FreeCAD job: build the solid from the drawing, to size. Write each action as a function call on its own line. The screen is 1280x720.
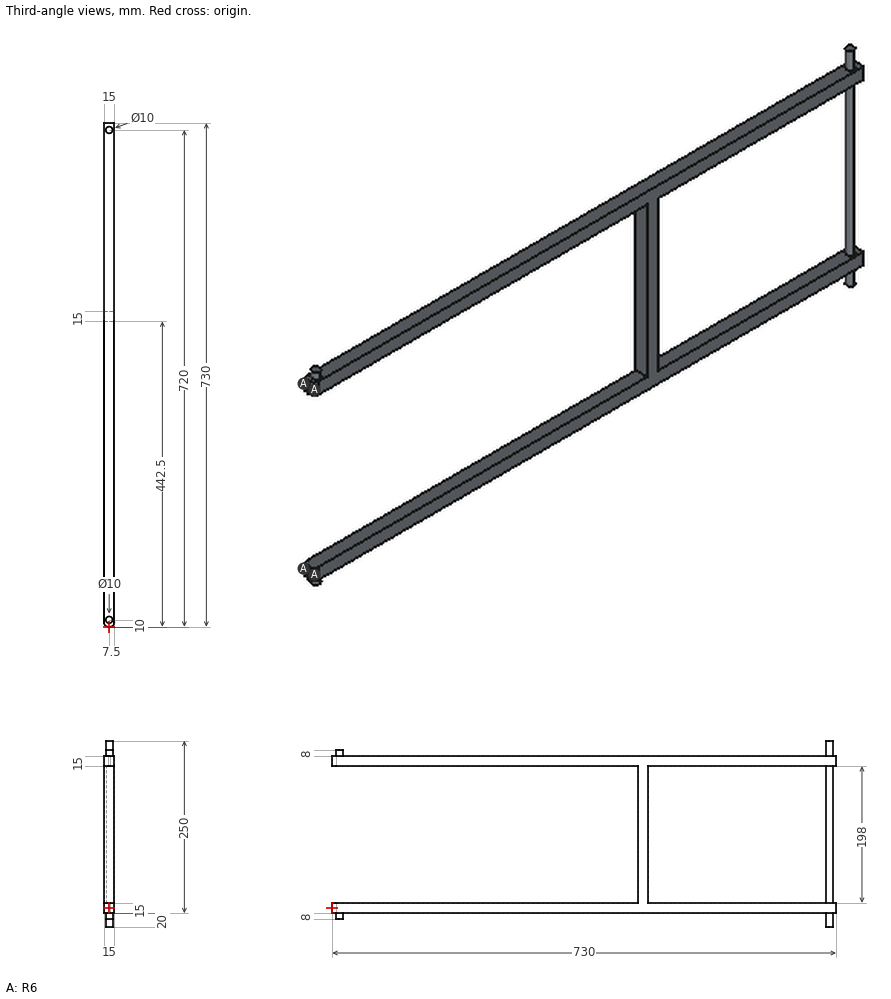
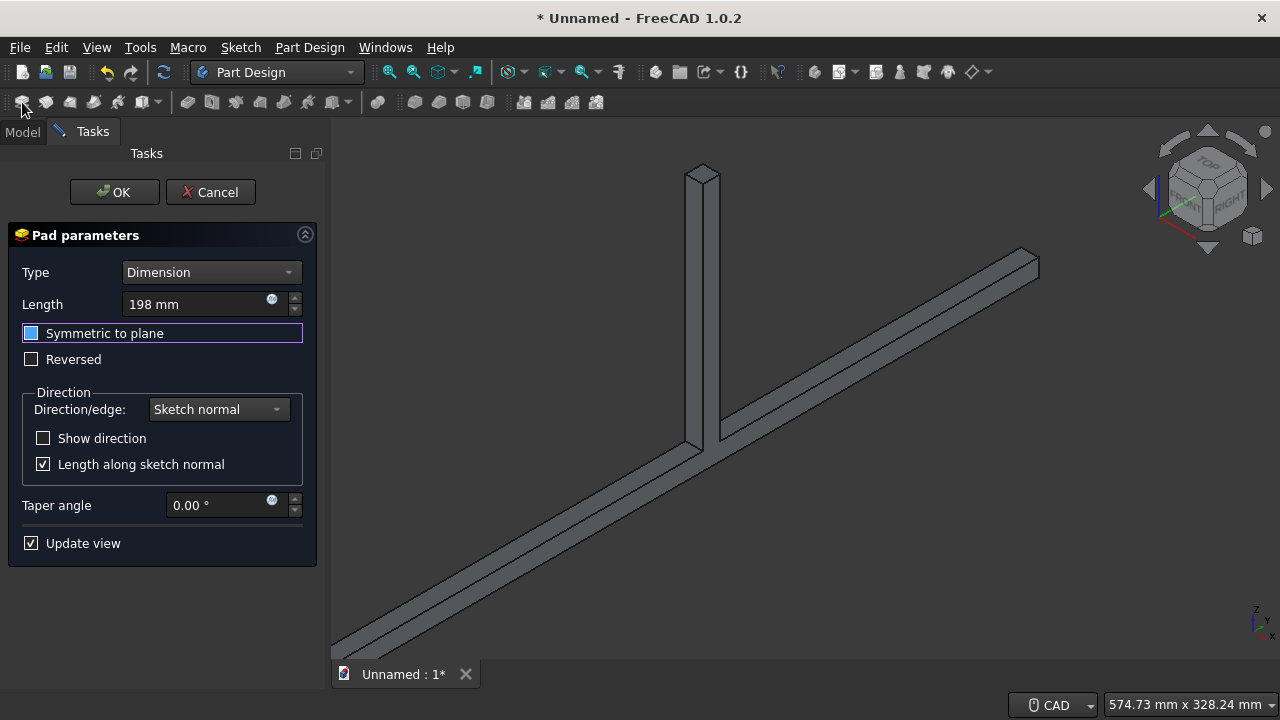
click(115, 192)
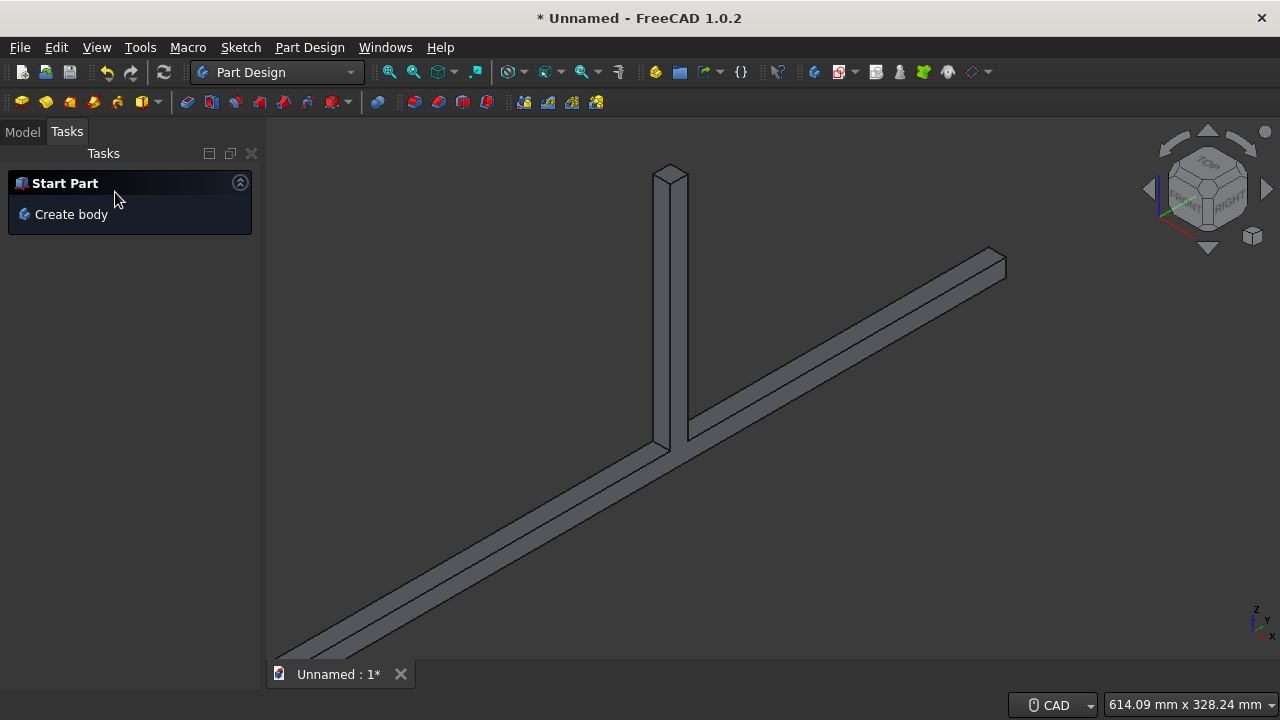
click(390, 72)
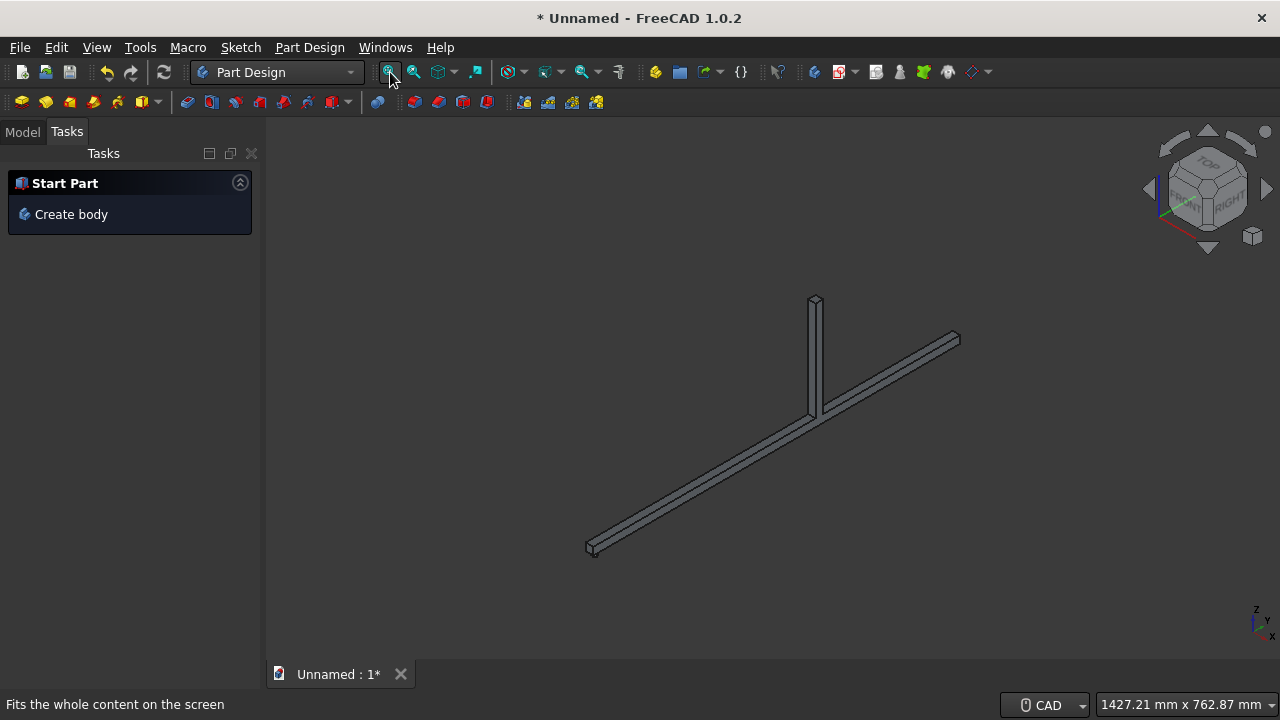
scroll(816, 298, up, 5)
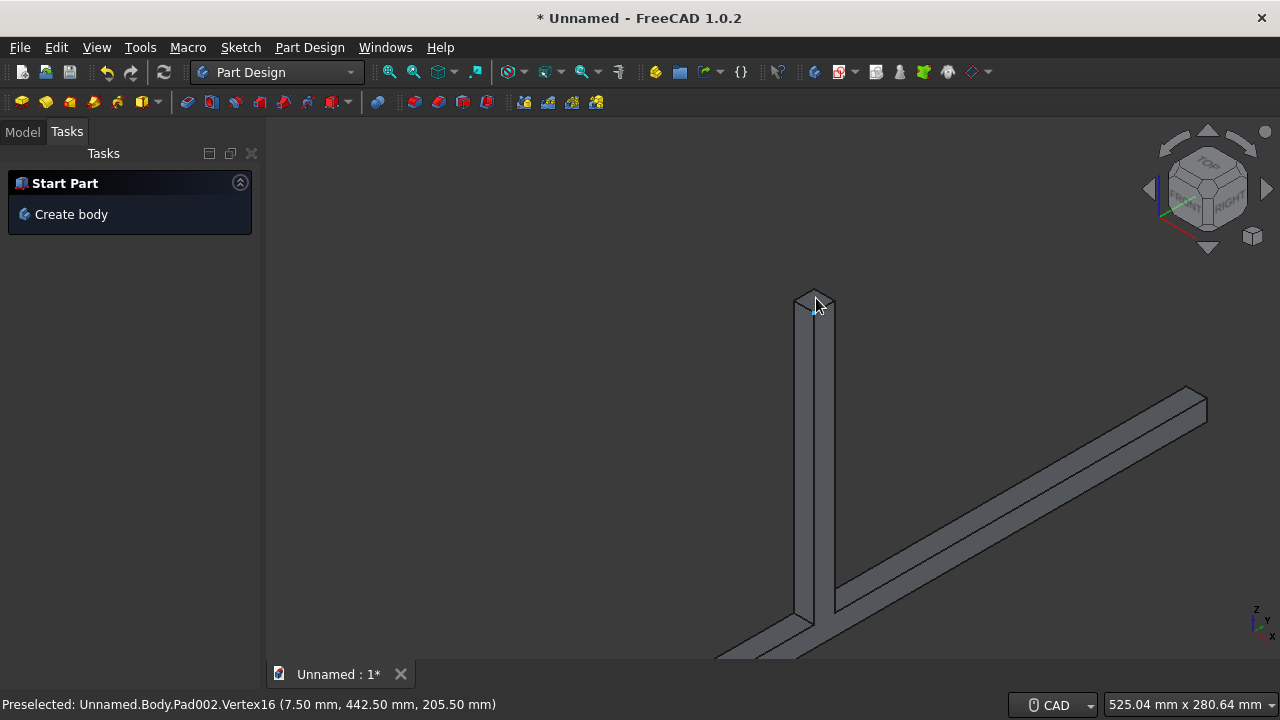
click(814, 300)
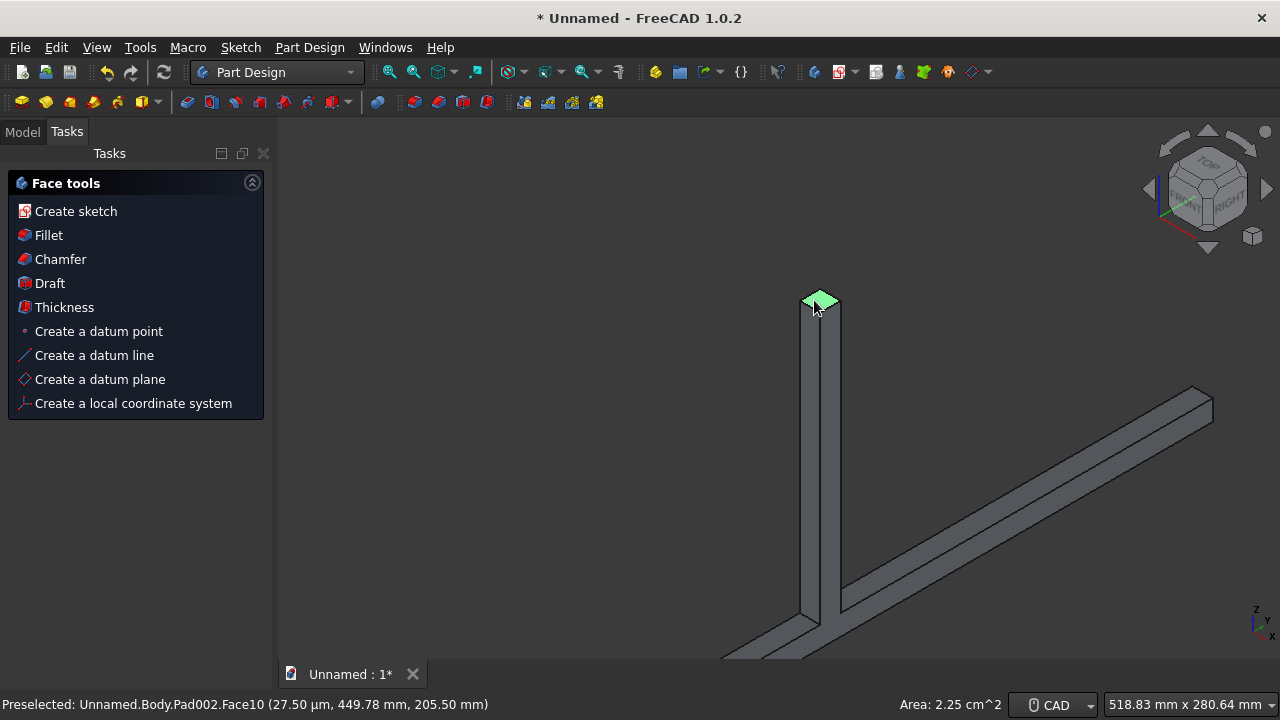
click(840, 72)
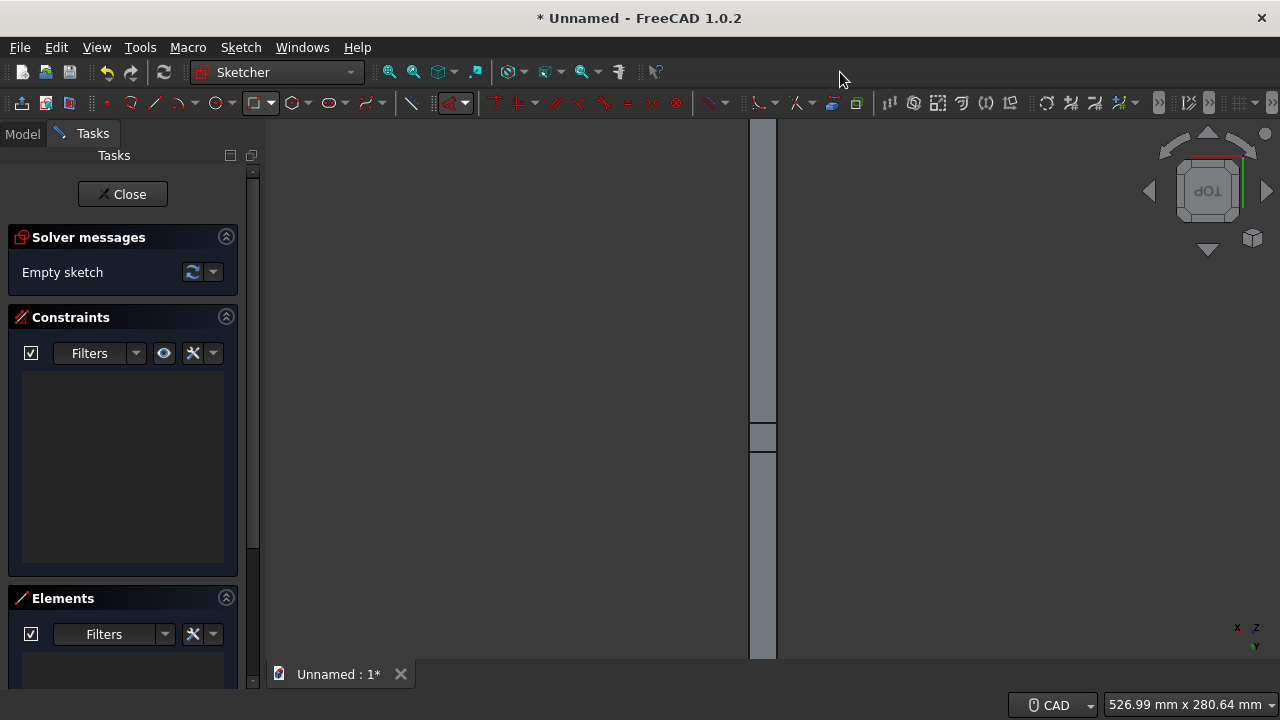
scroll(685, 427, down, 7)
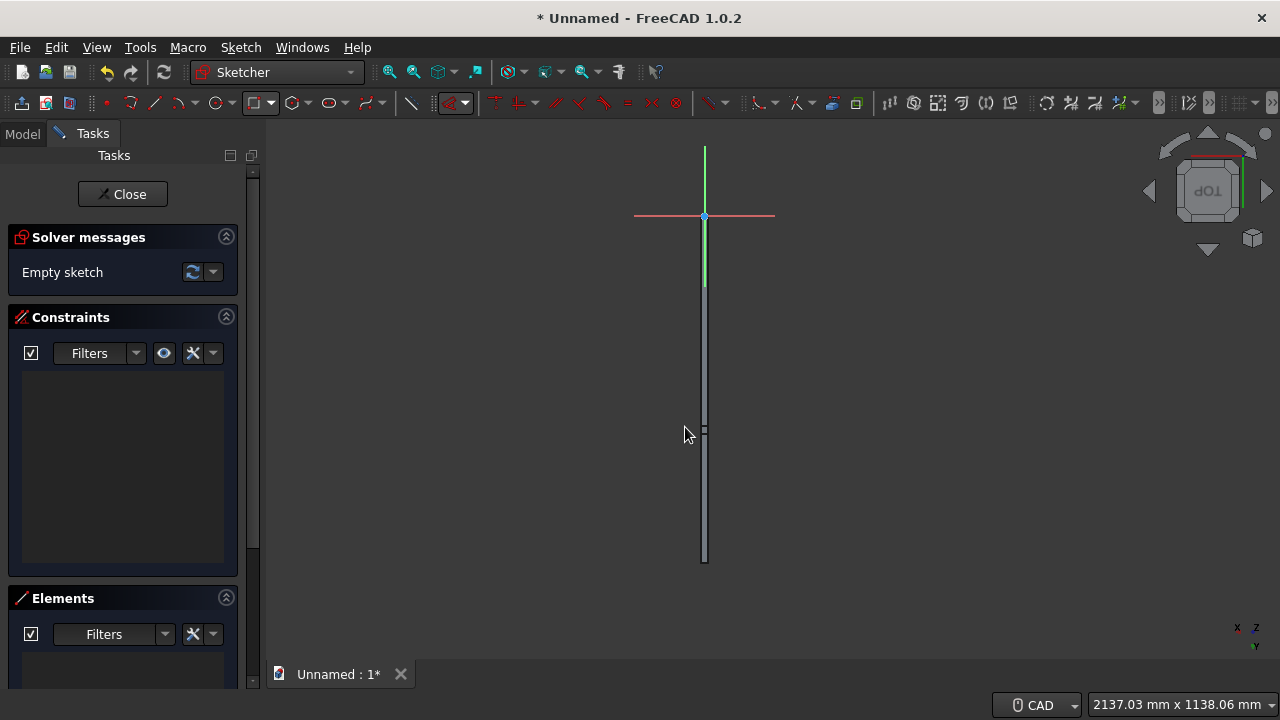
click(254, 104)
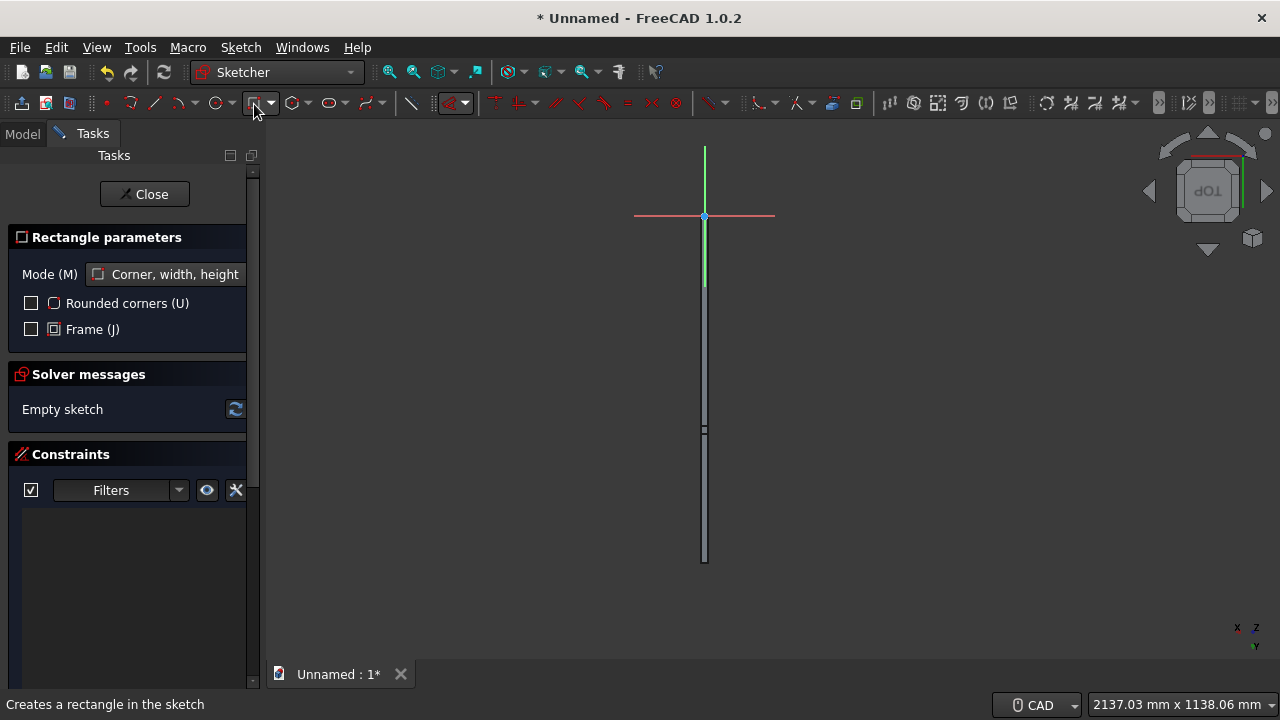
scroll(701, 216, up, 8)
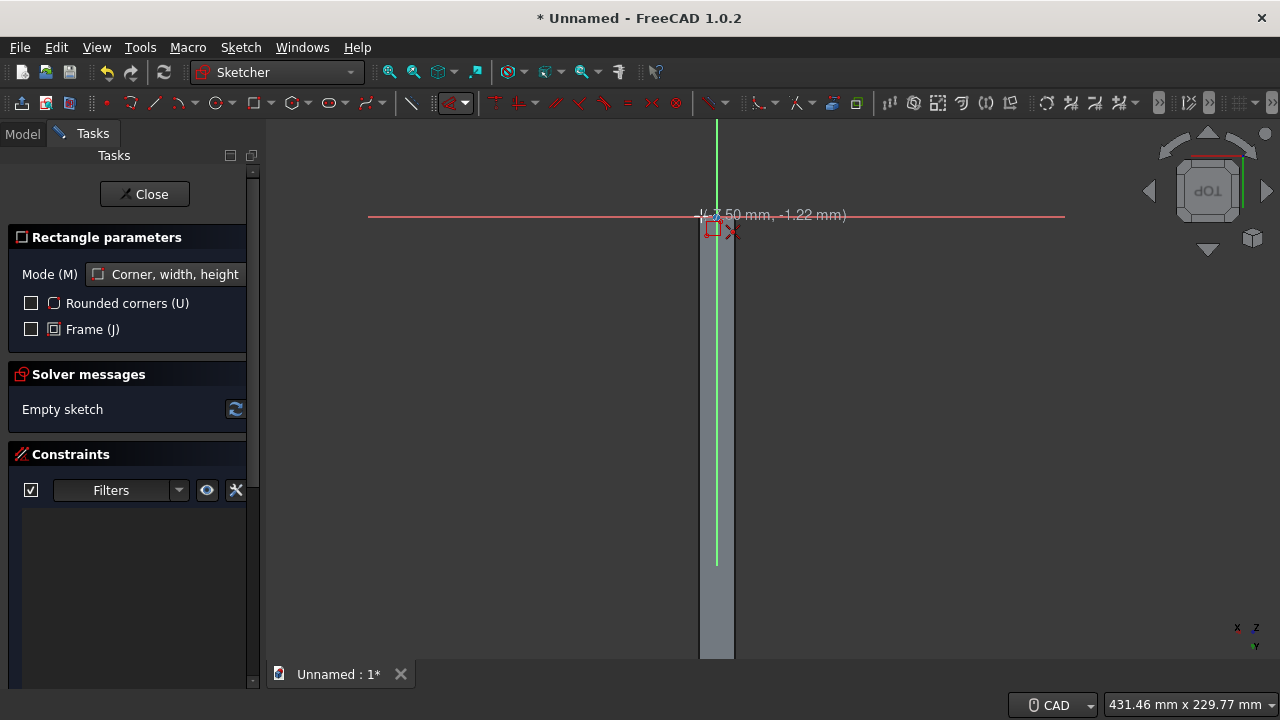
click(699, 217)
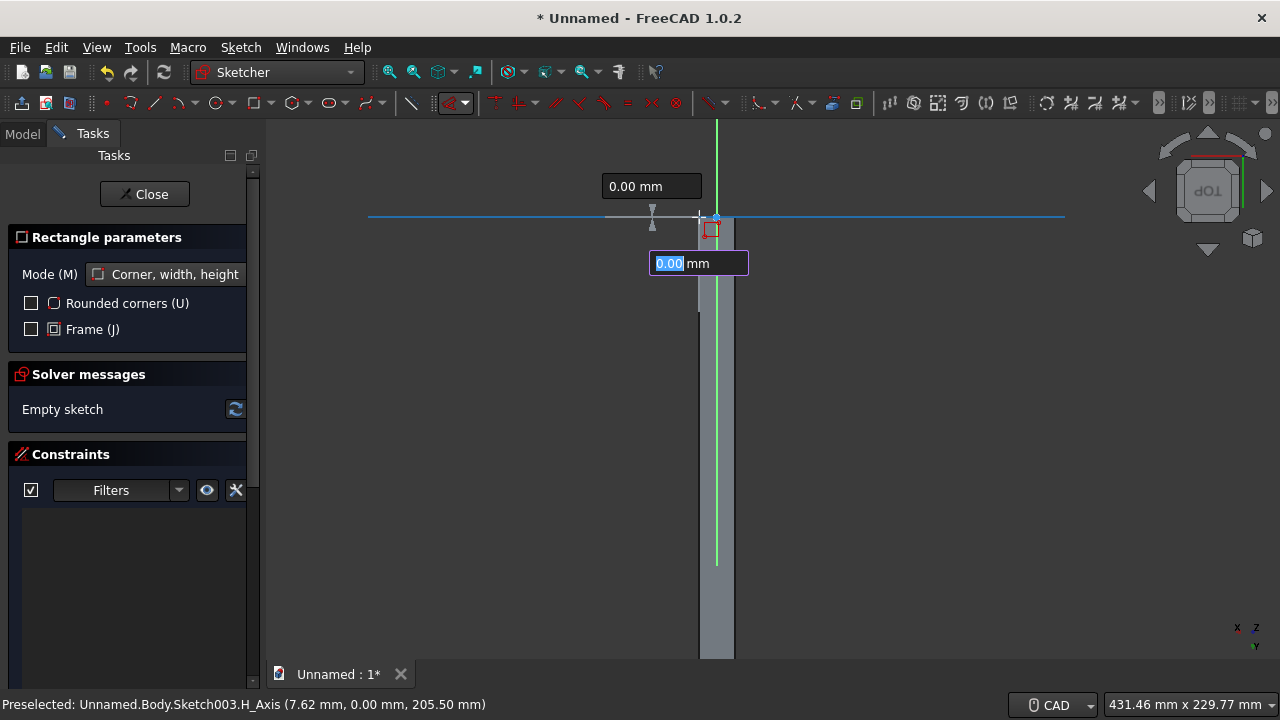
scroll(701, 215, down, 8)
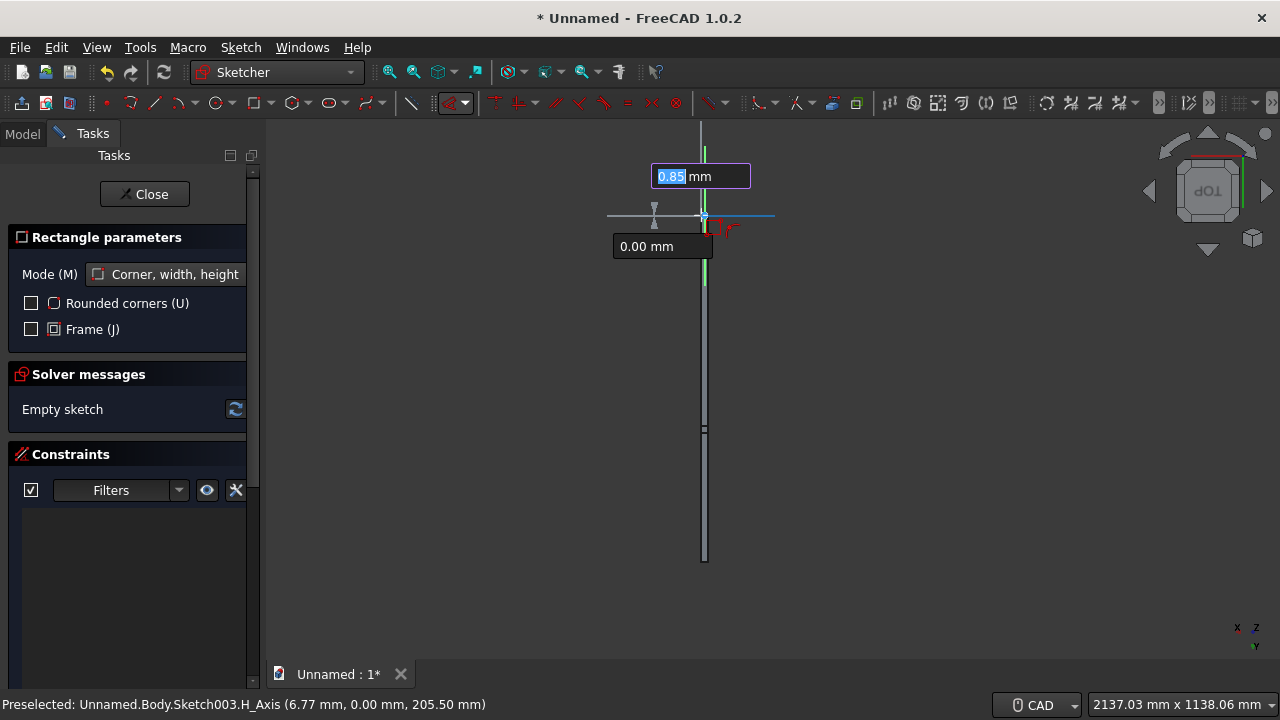
scroll(708, 562, up, 8)